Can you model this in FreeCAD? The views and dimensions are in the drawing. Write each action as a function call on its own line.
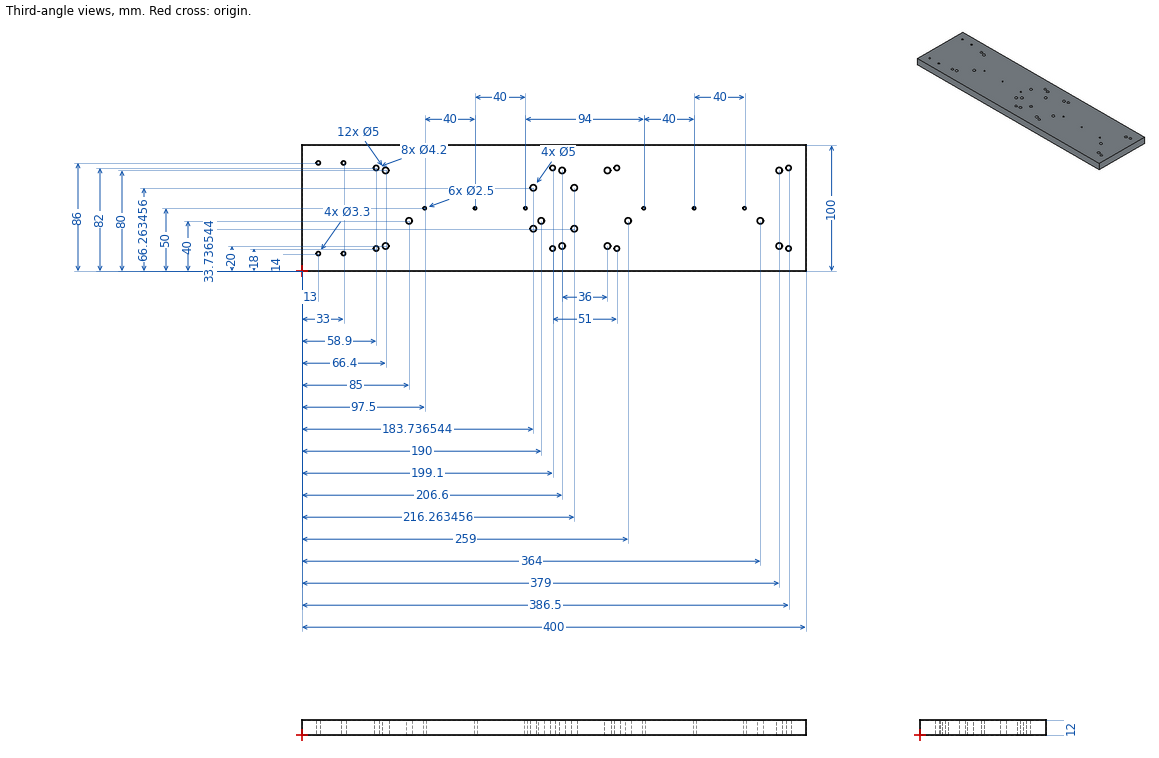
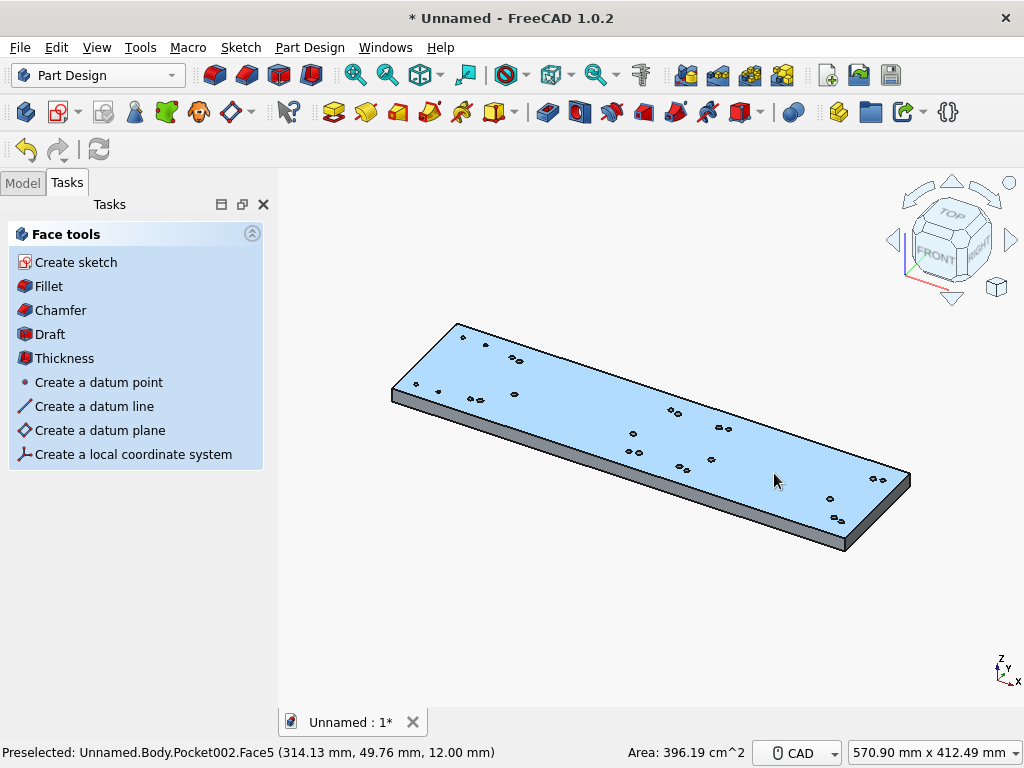
click(58, 112)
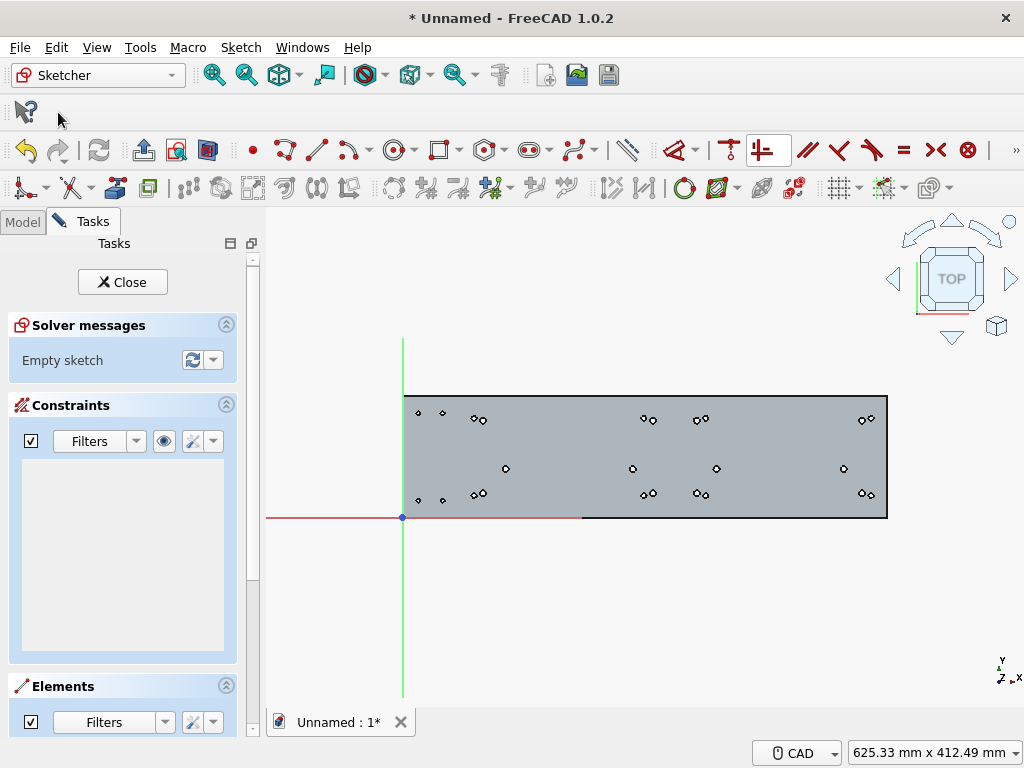
scroll(656, 457, up, 10)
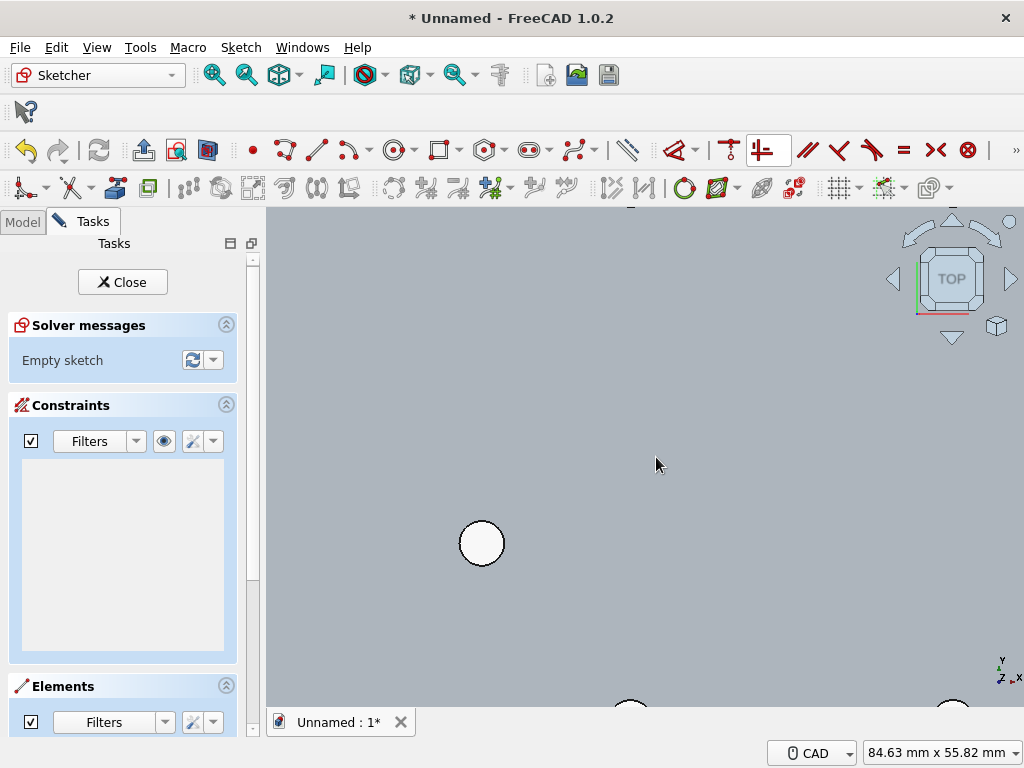
click(394, 150)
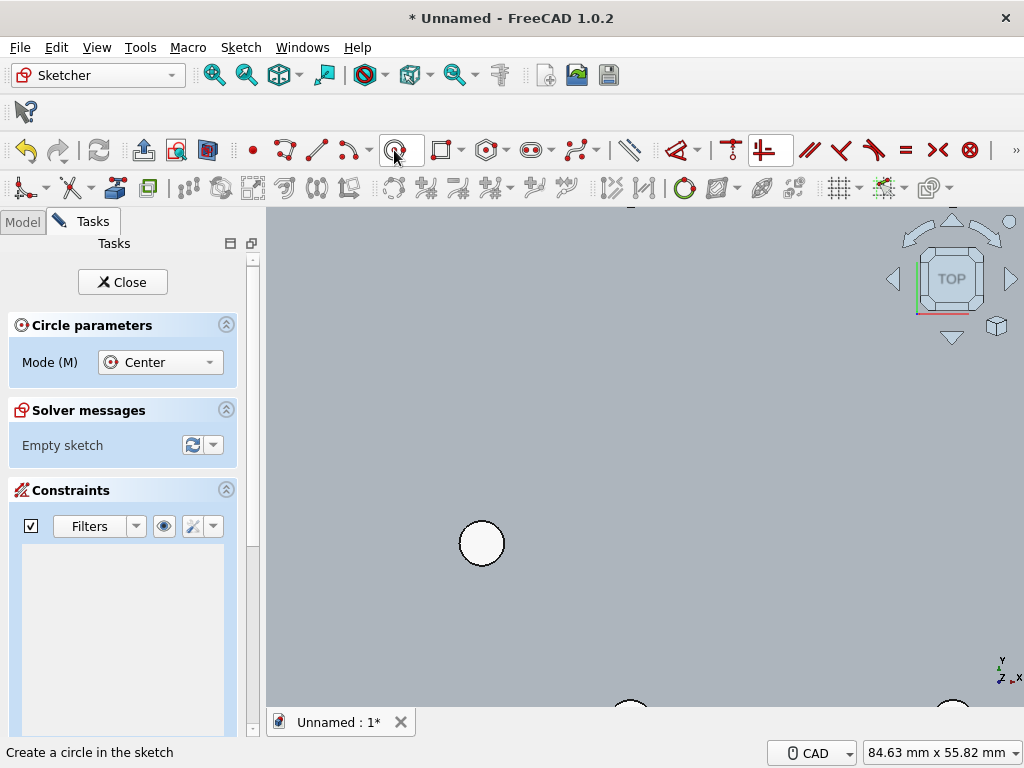
click(426, 308)
click(442, 292)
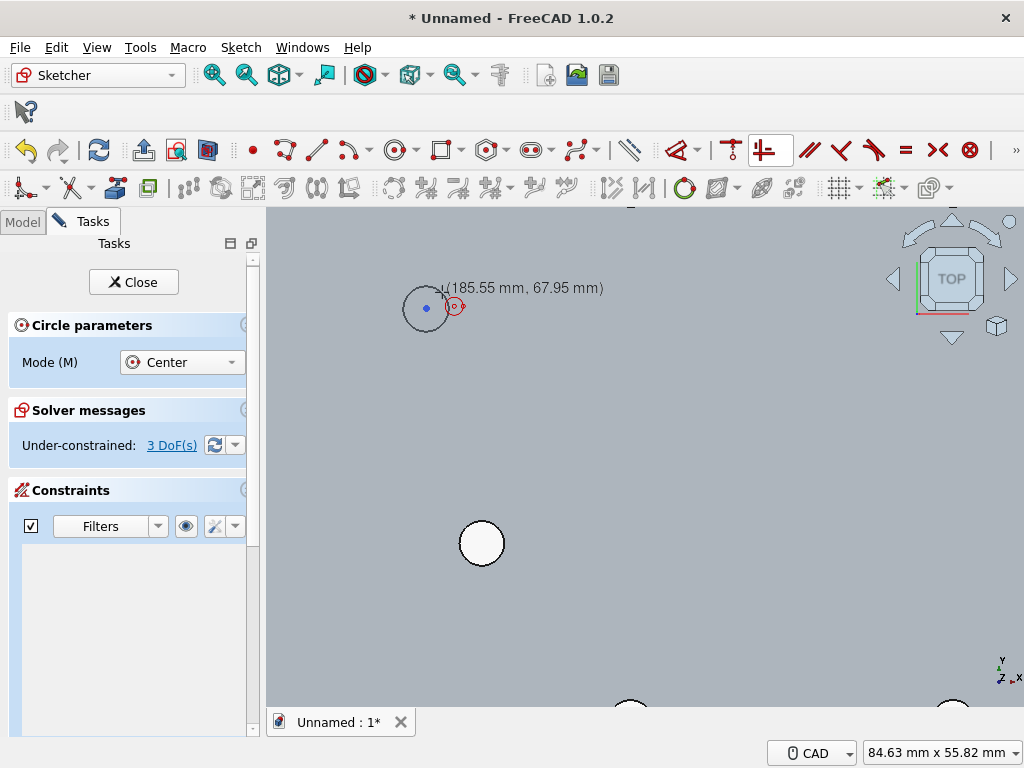
click(717, 308)
click(733, 292)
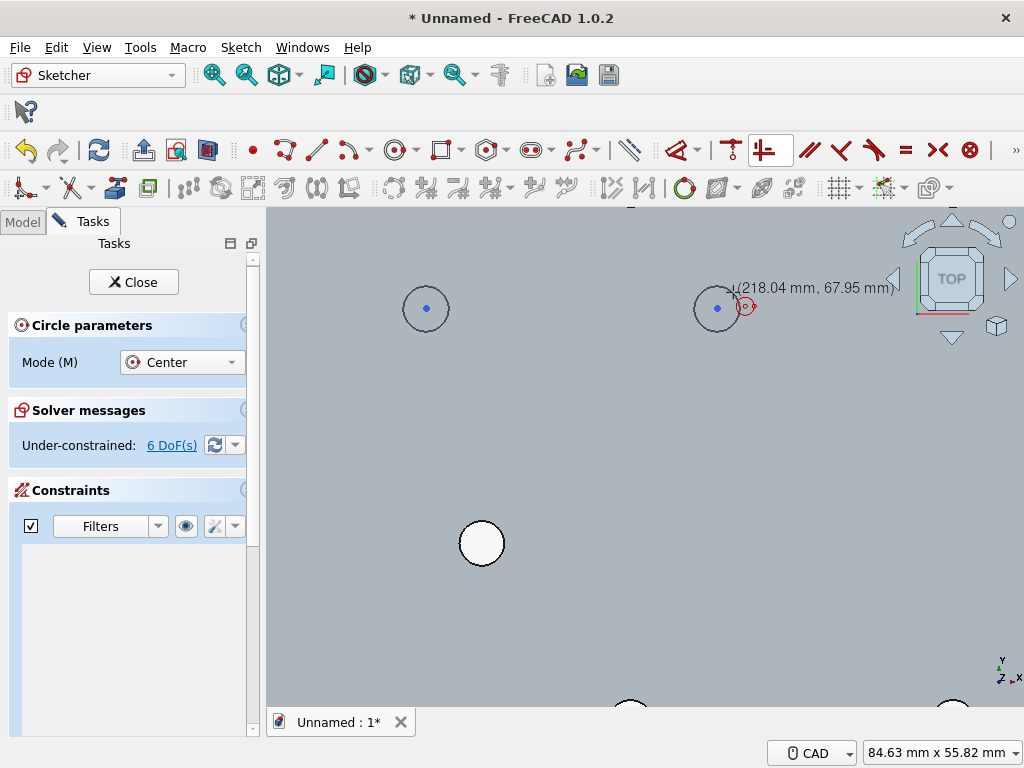
click(717, 599)
click(733, 584)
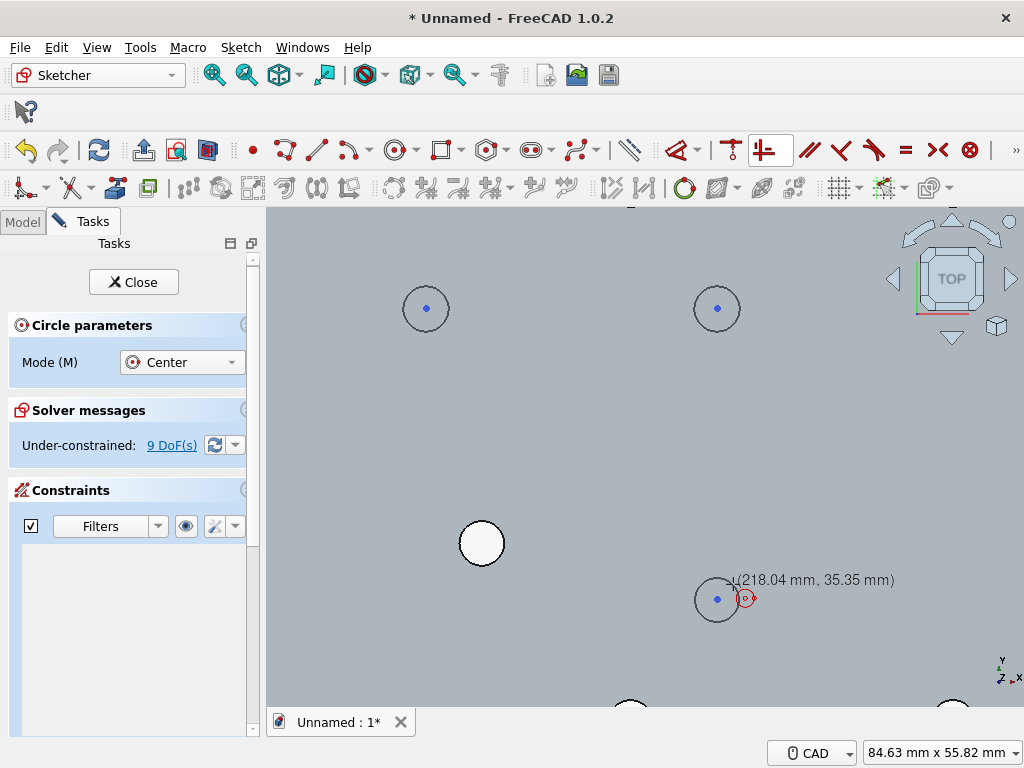
click(426, 599)
click(442, 584)
key(Escape)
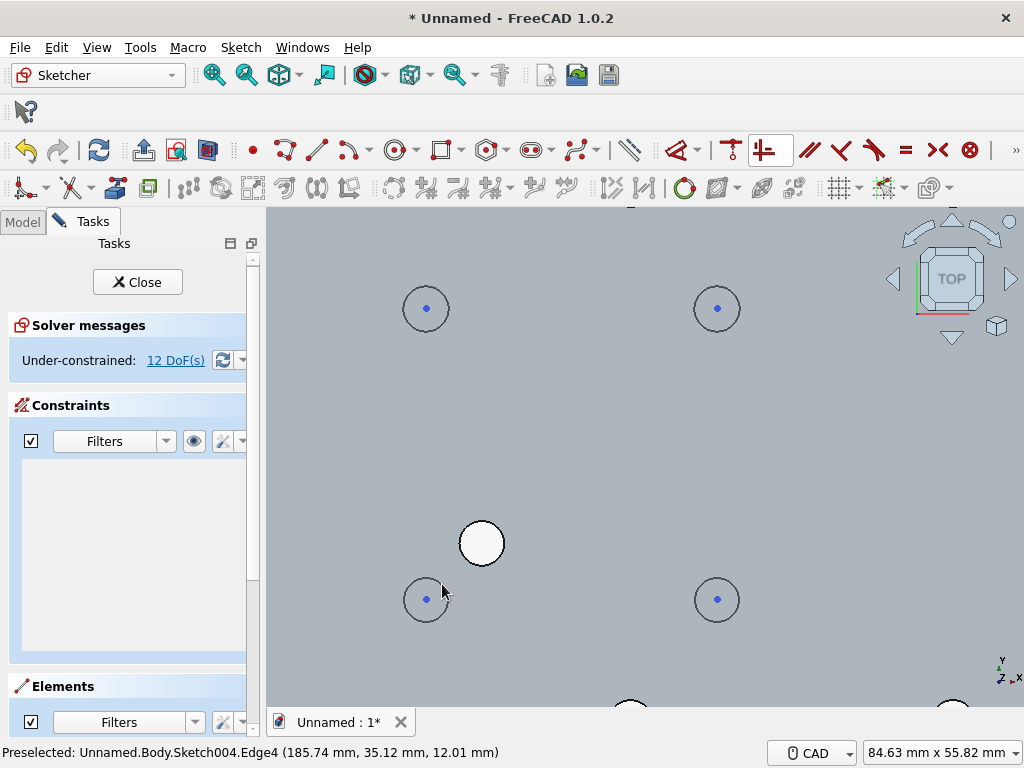
click(442, 293)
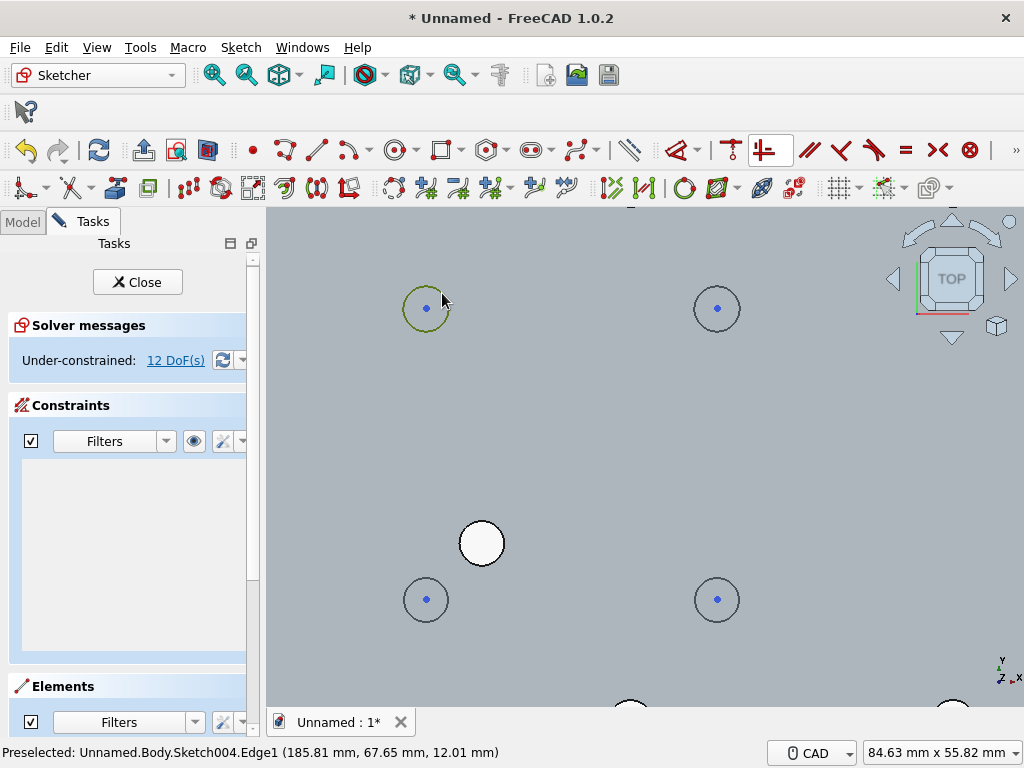
click(733, 293)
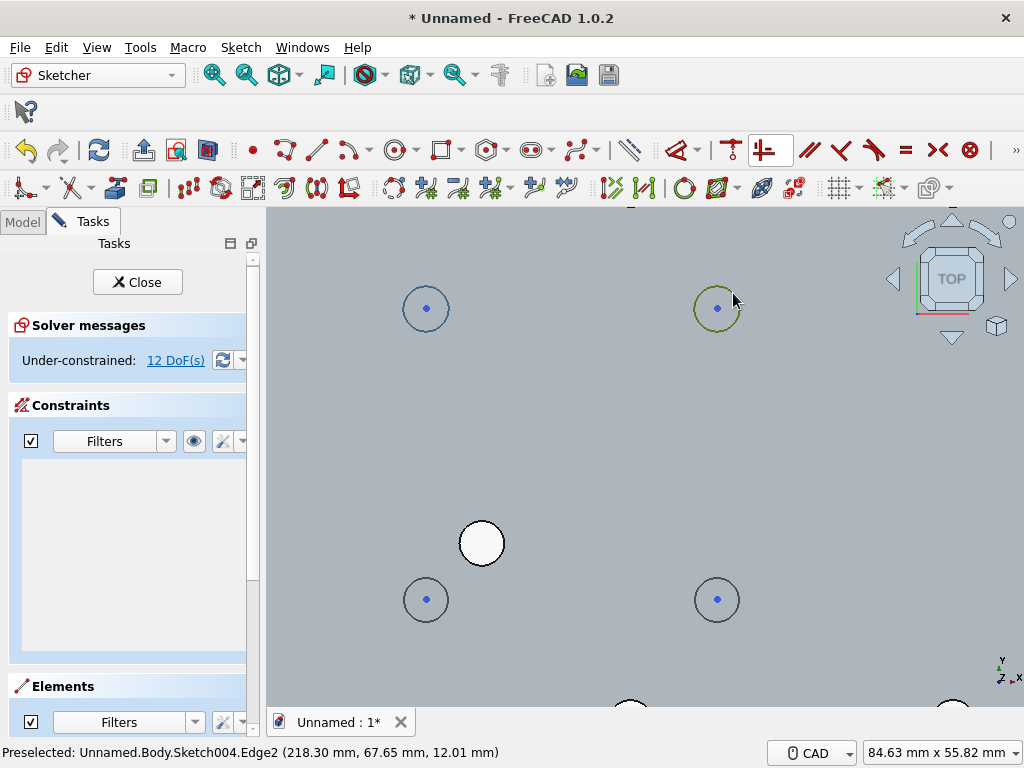
click(732, 584)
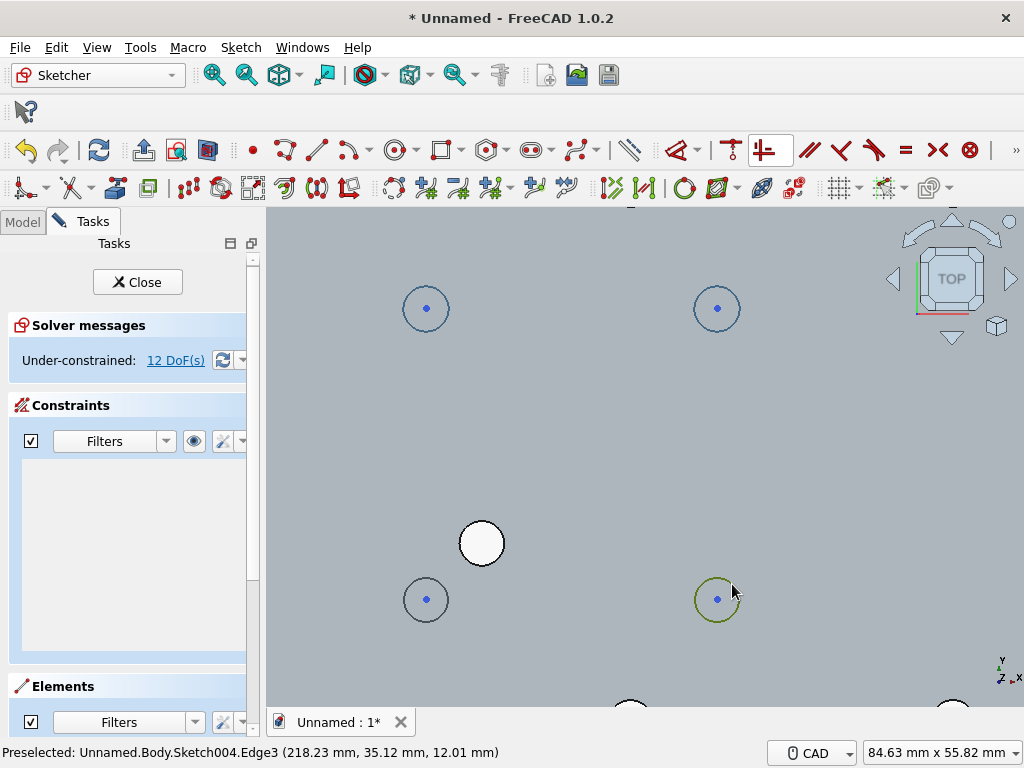
click(441, 584)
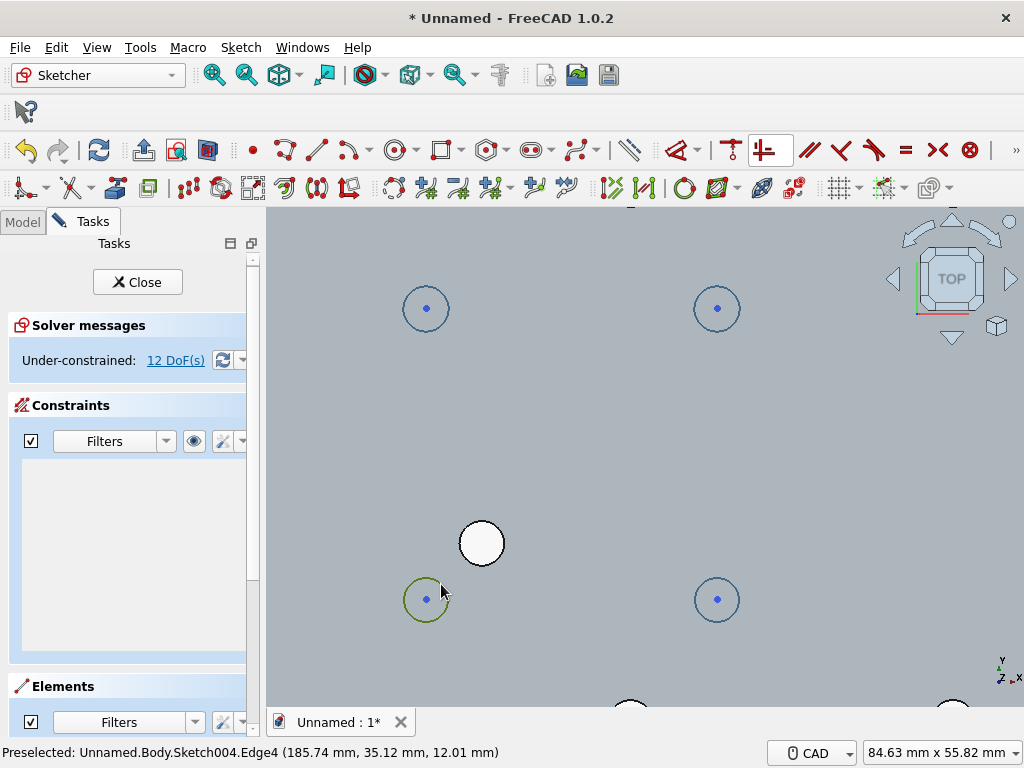
click(906, 150)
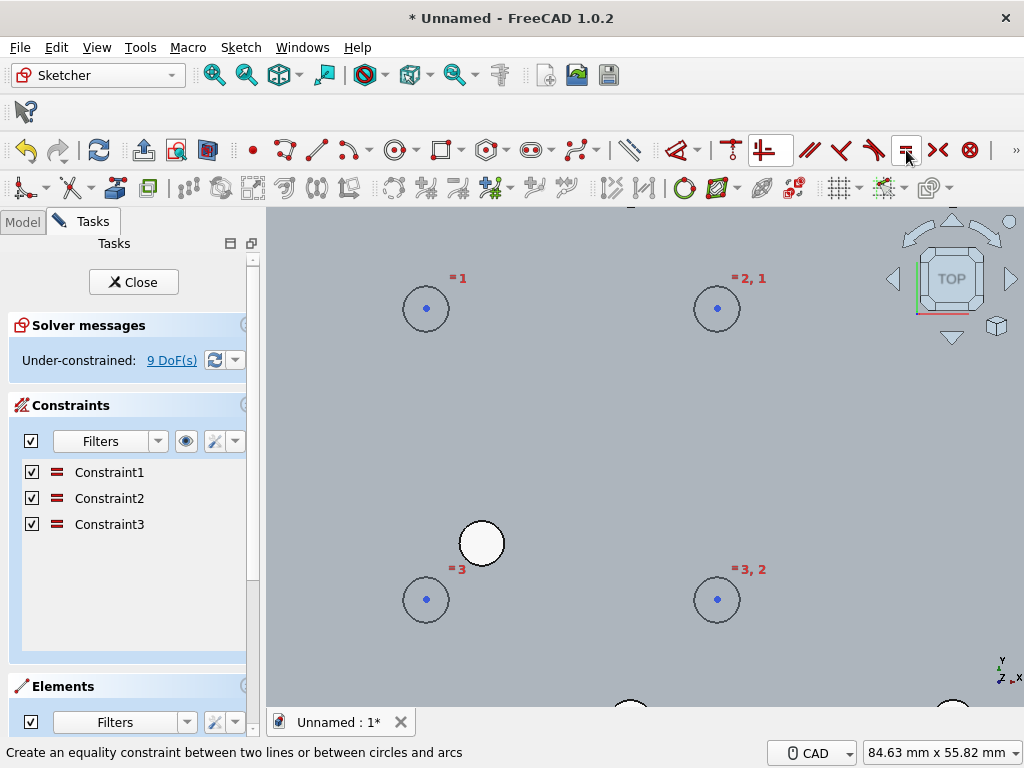
click(426, 309)